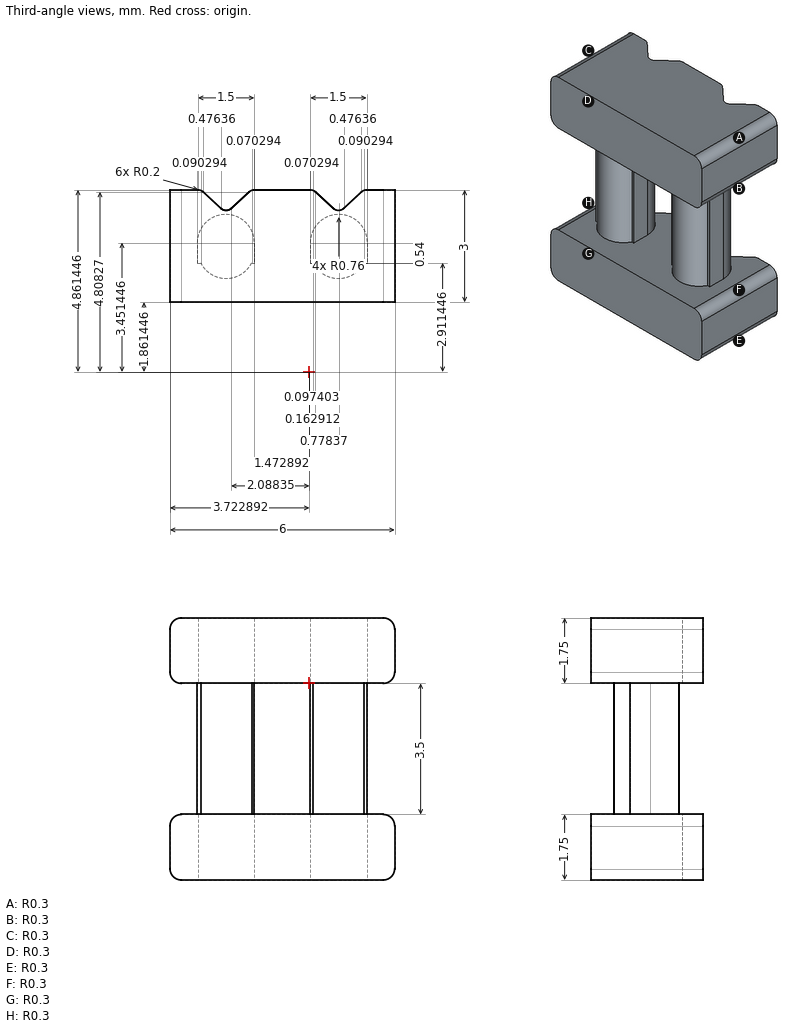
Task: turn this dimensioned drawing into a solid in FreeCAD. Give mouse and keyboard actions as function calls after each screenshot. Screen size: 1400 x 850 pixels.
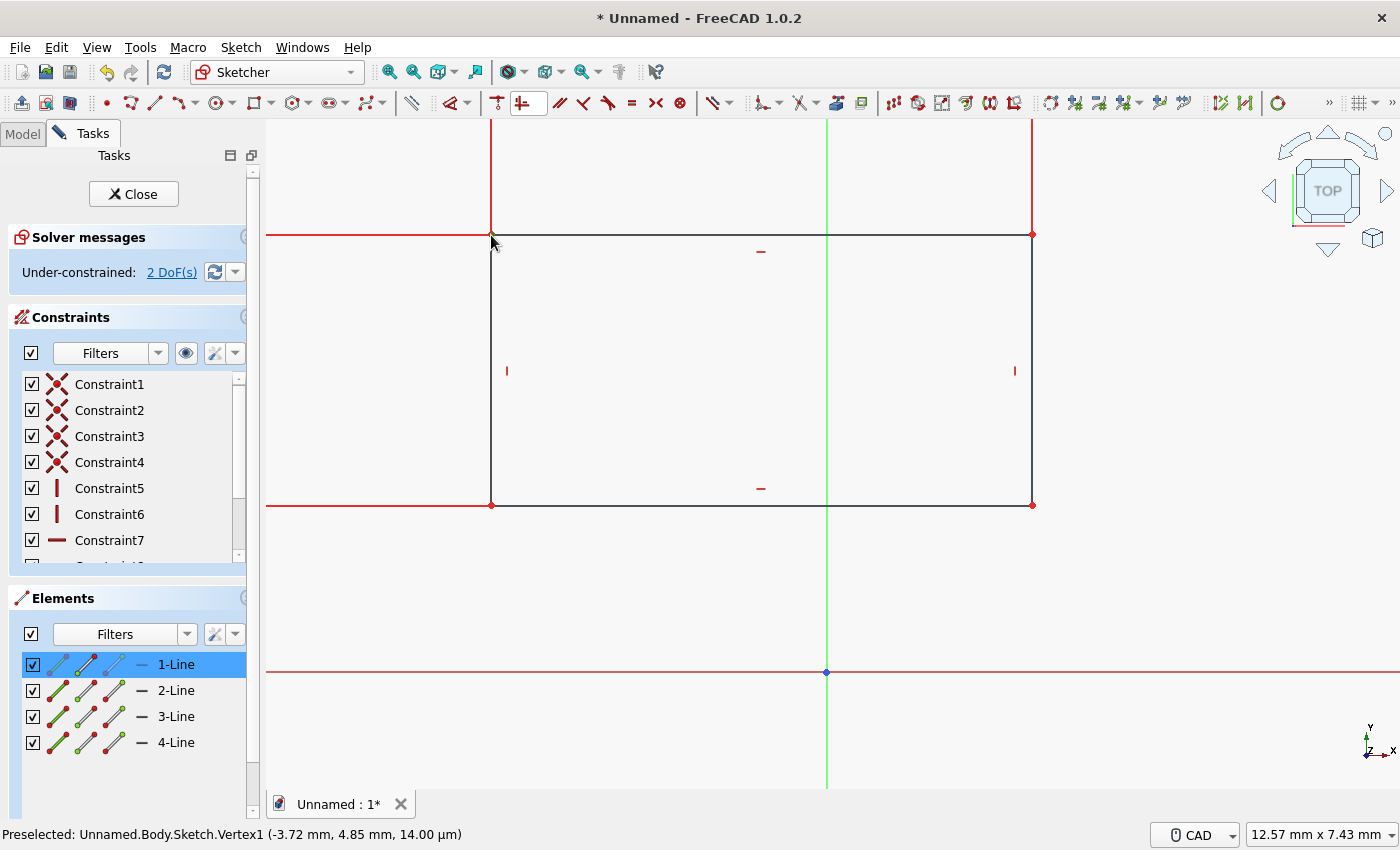
click(470, 104)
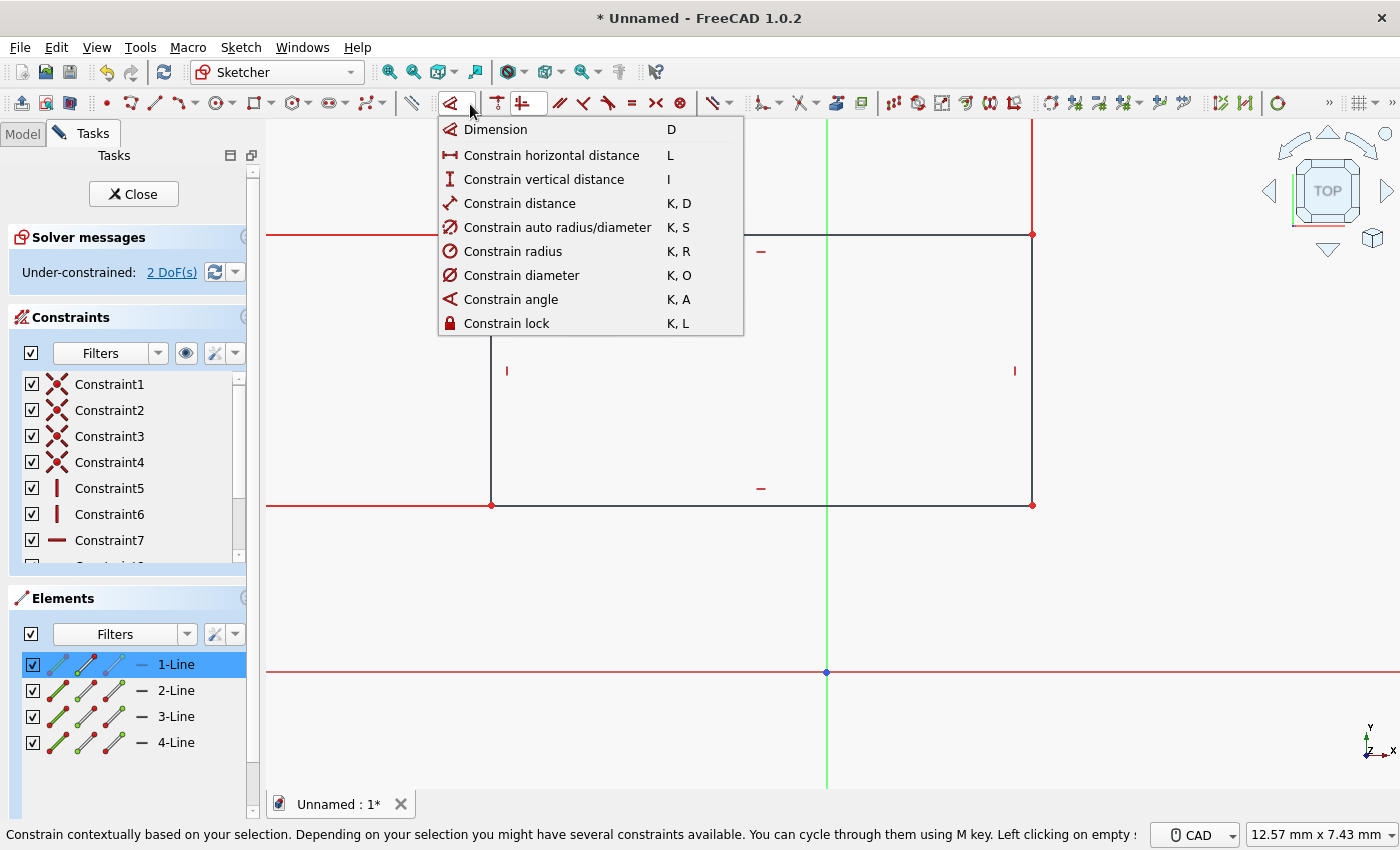
click(591, 155)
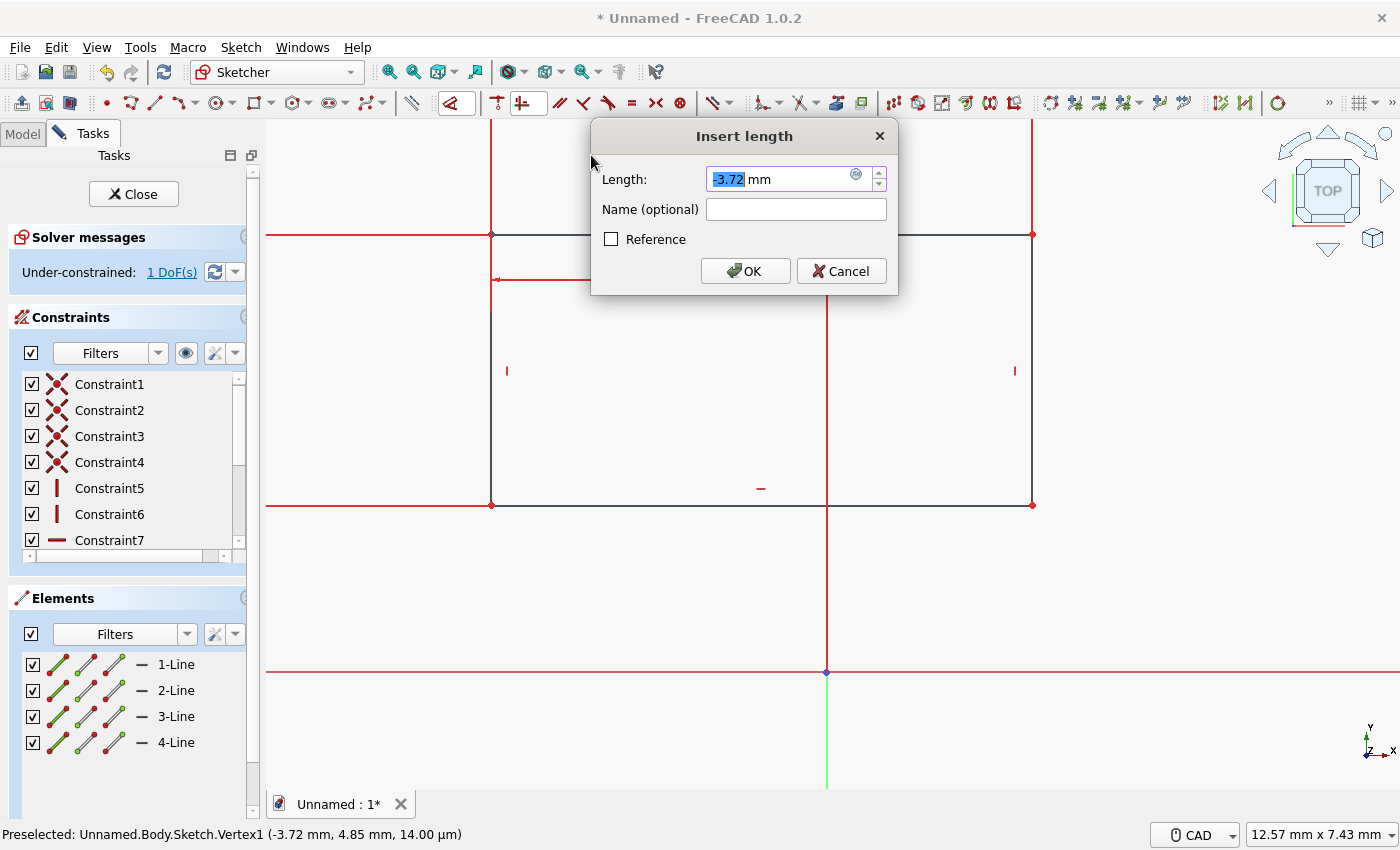
text(-3.722892)
key(Return)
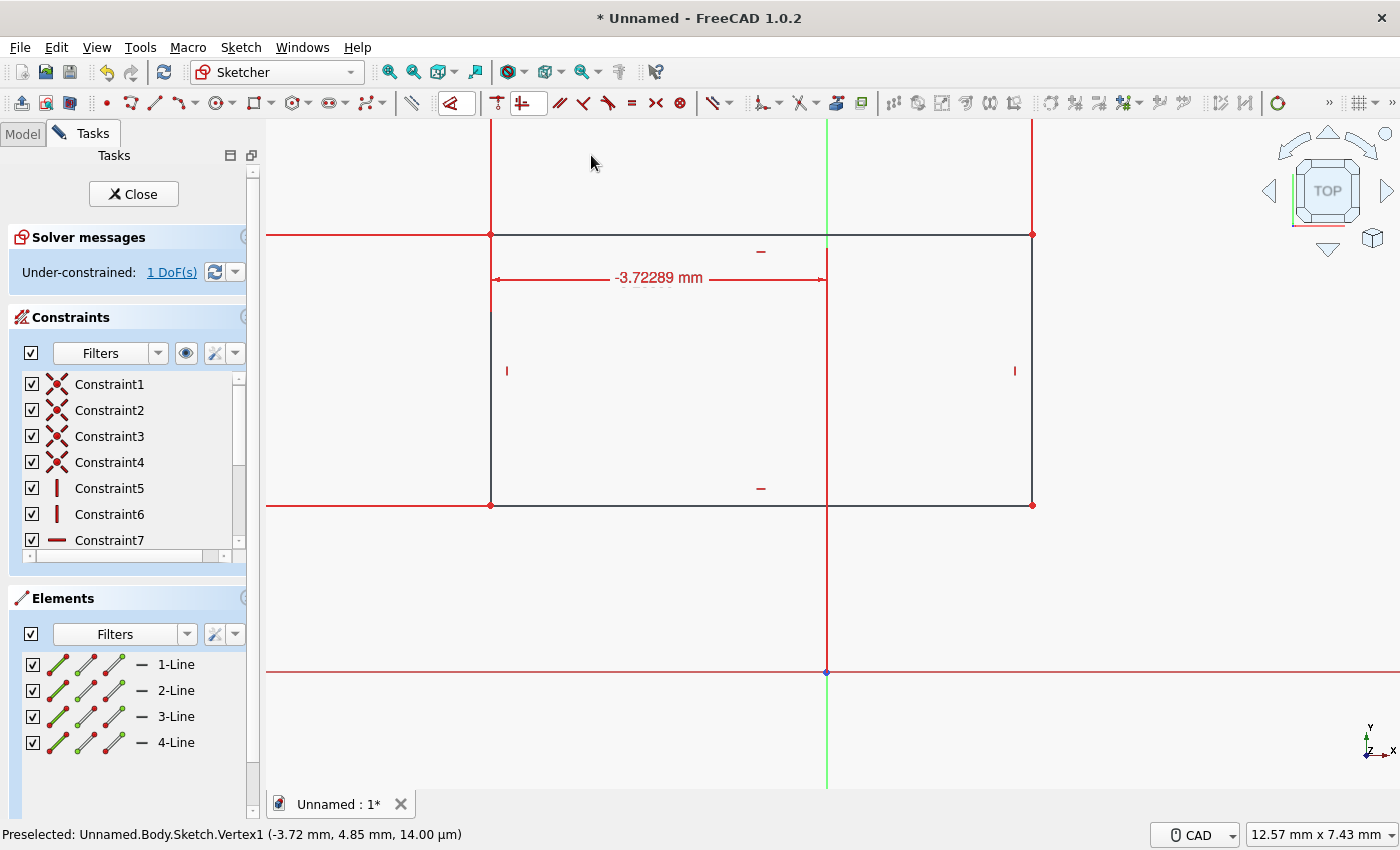
click(491, 235)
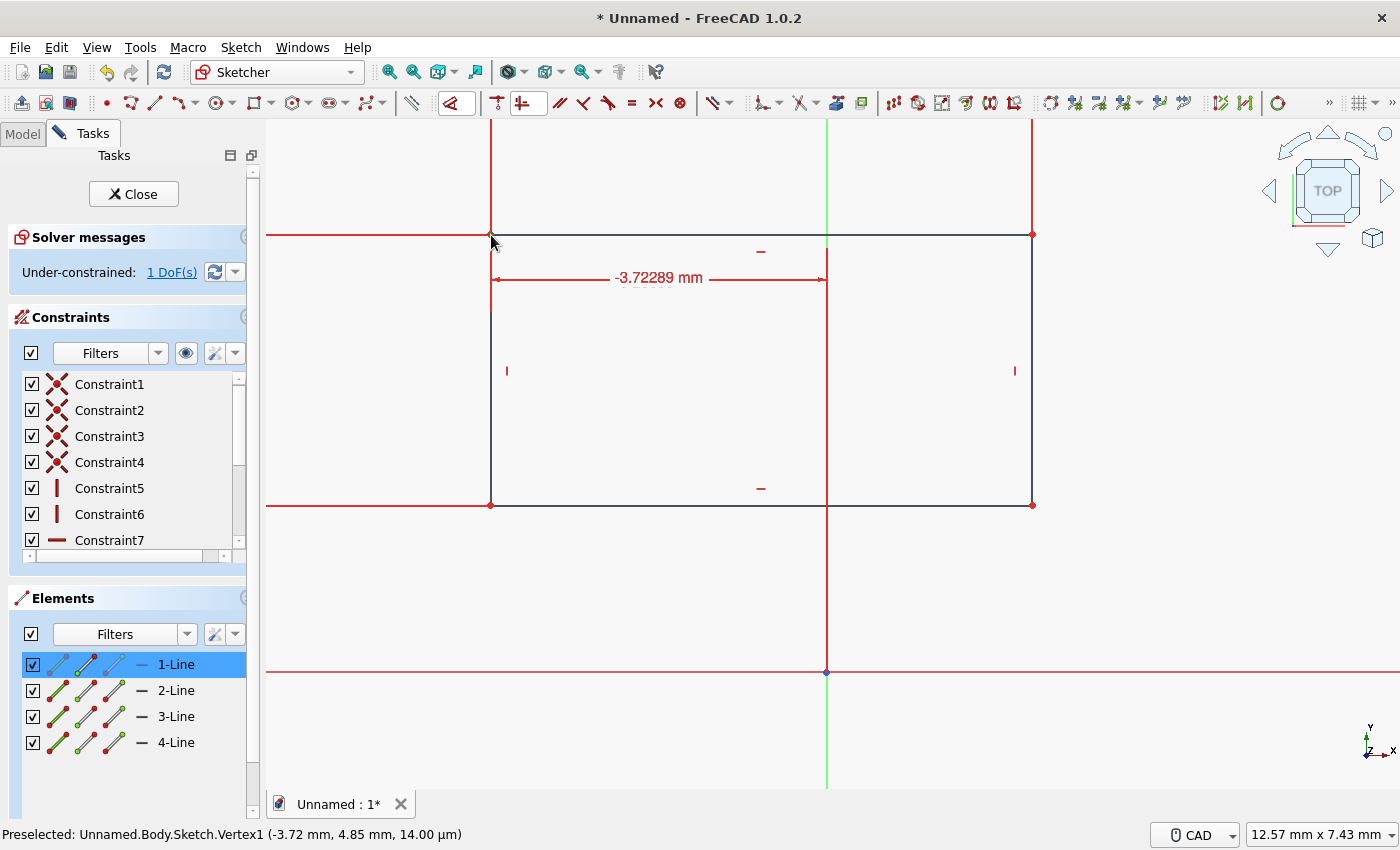
key(i)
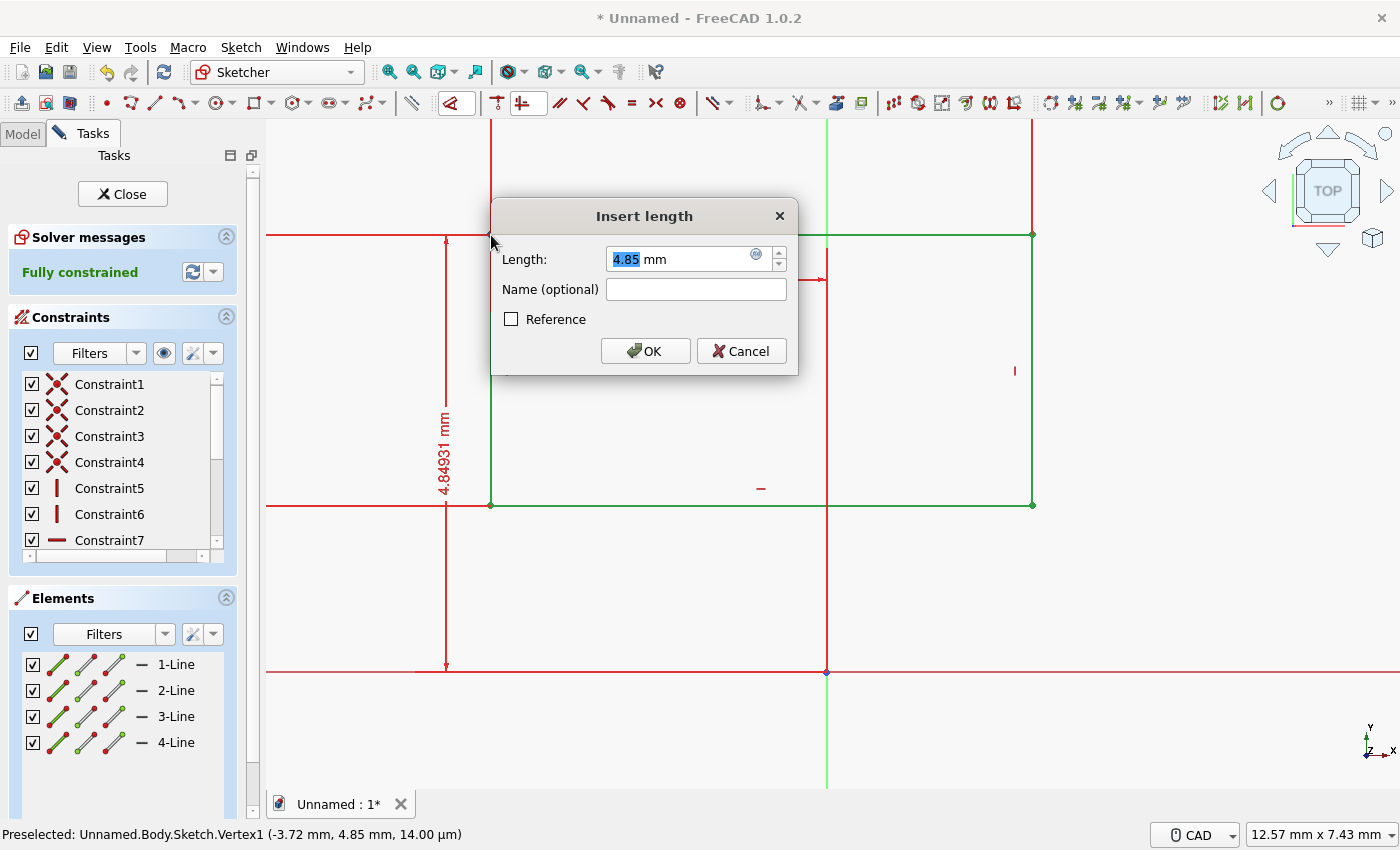
text(4.861446)
key(Return)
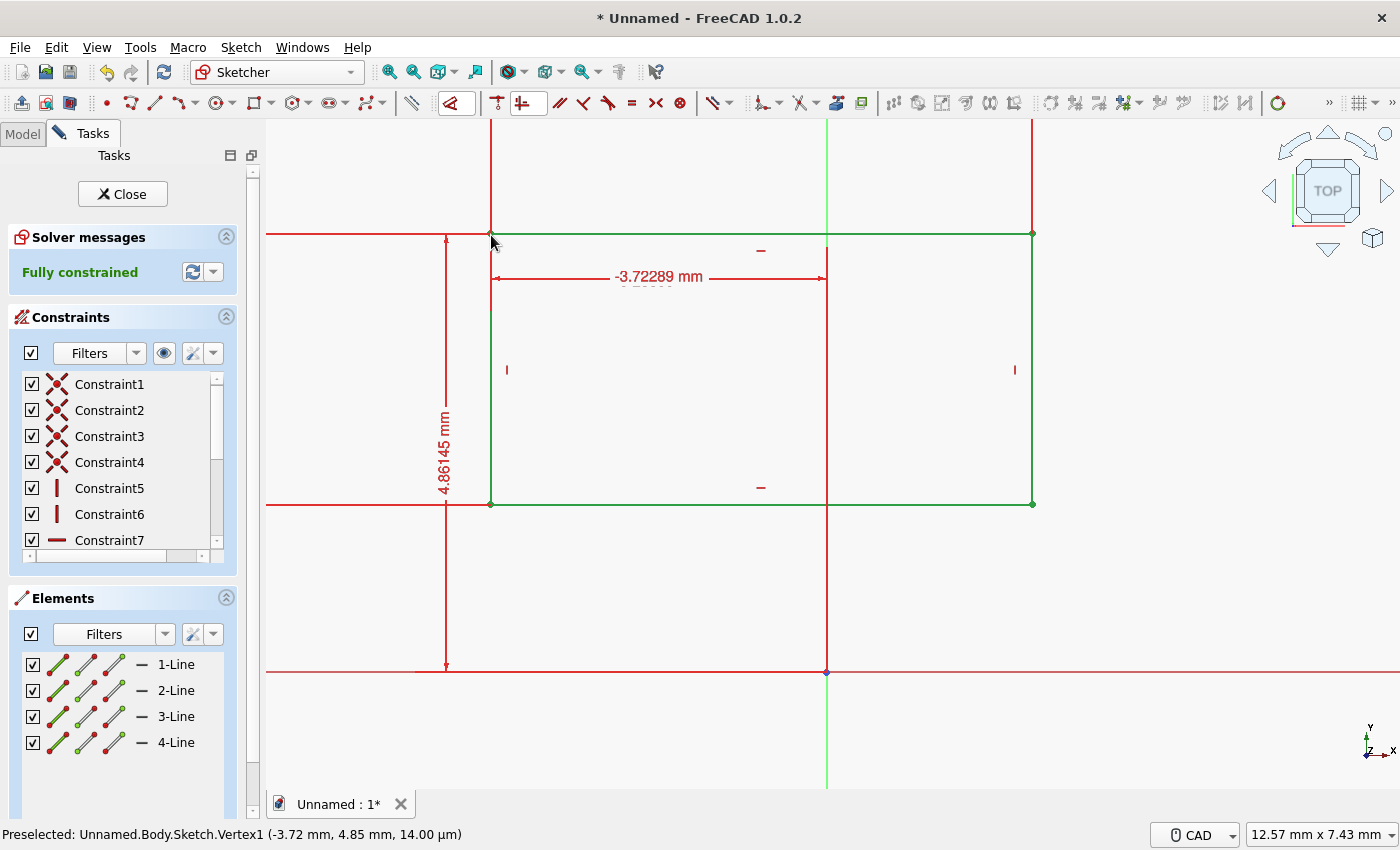
click(123, 194)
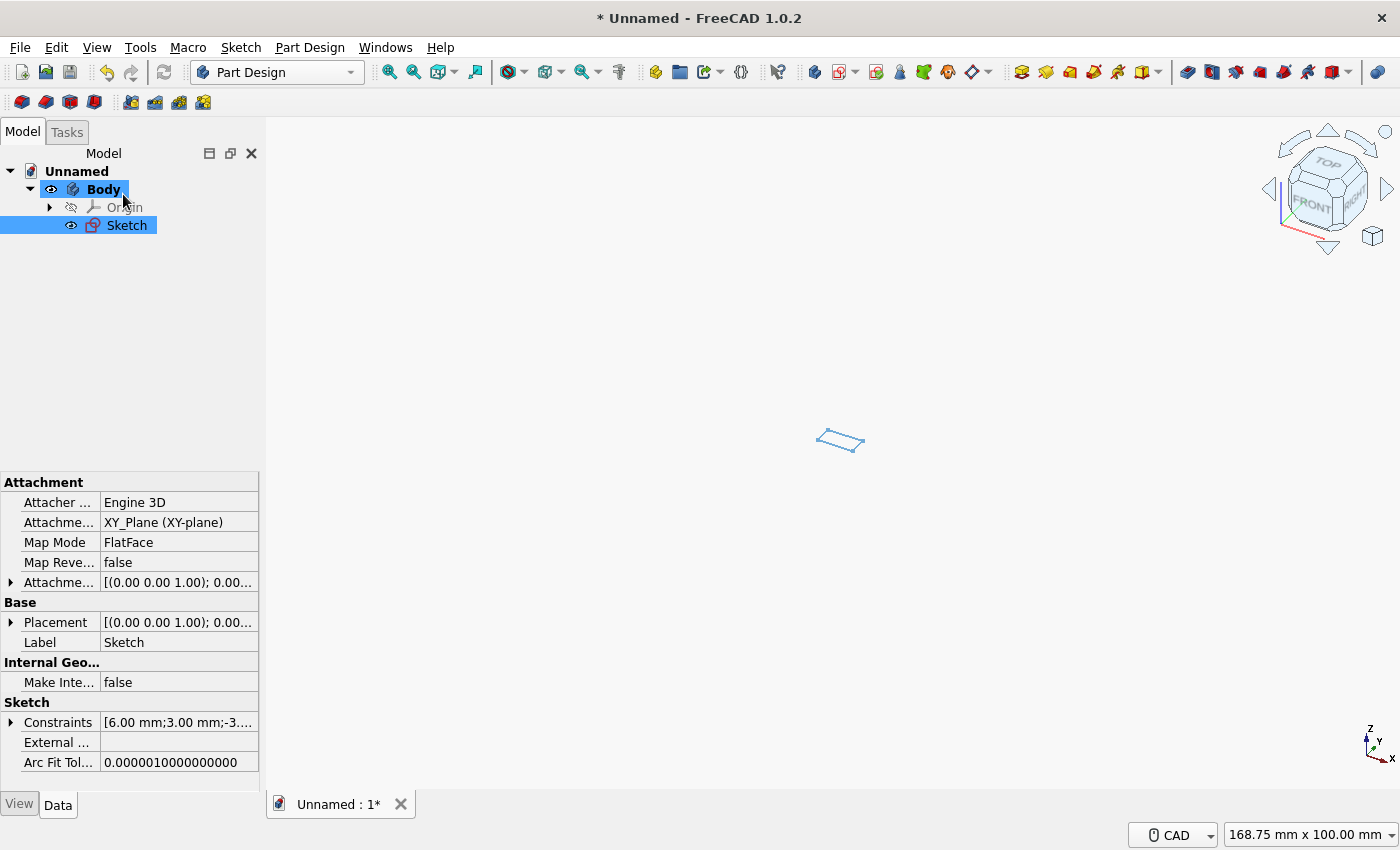
click(1022, 72)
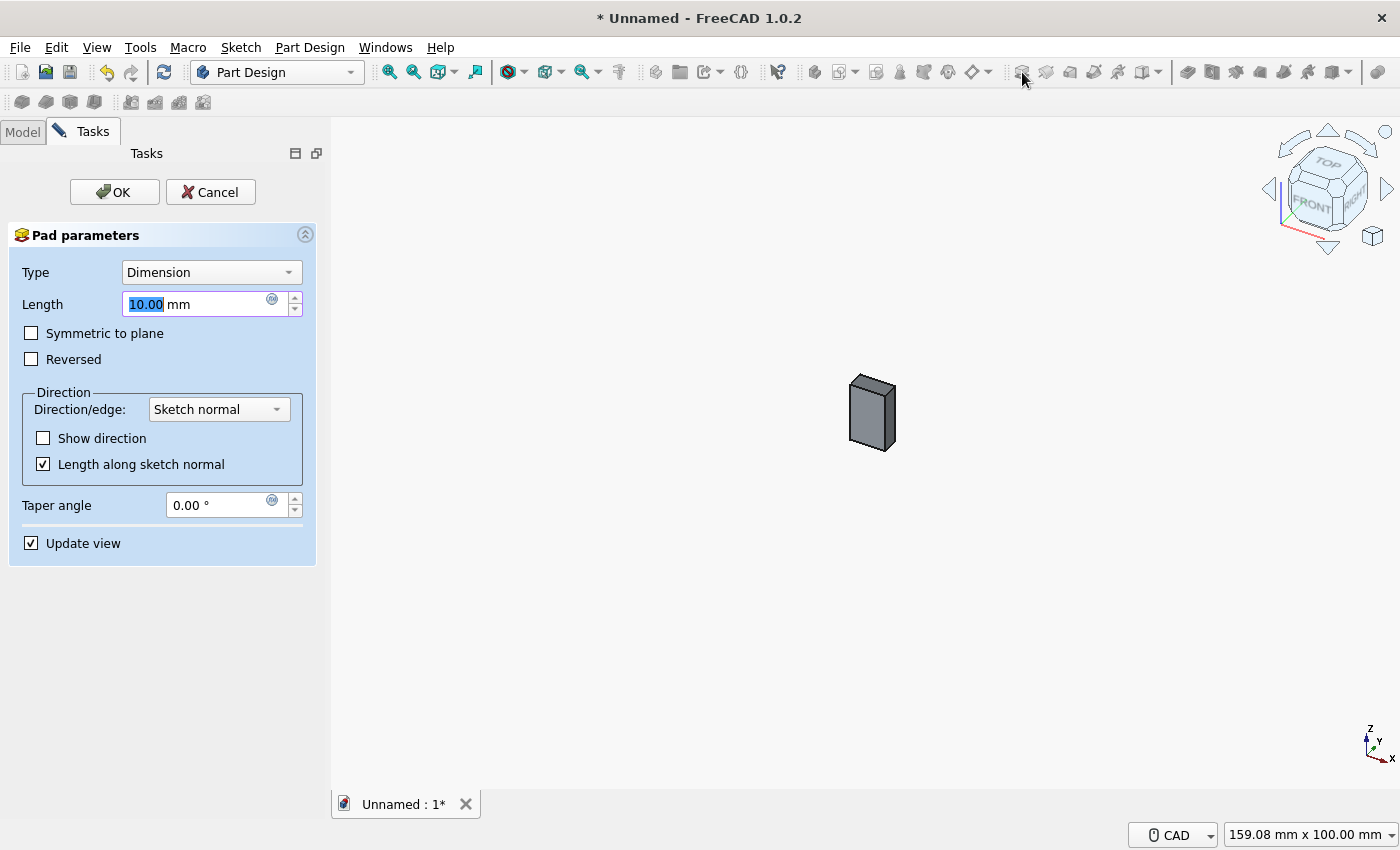
text(1.75)
key(Tab)